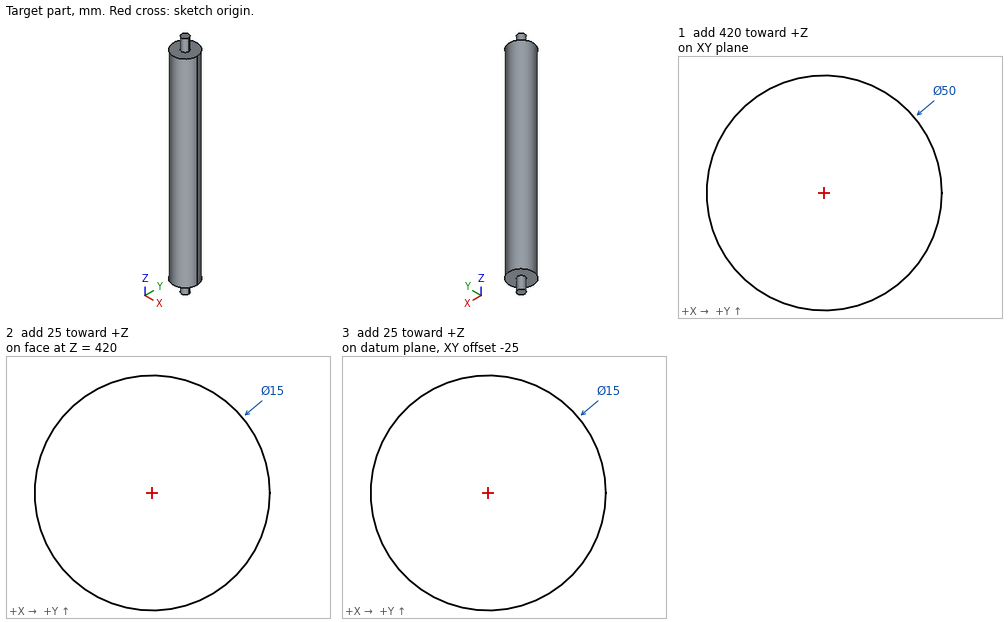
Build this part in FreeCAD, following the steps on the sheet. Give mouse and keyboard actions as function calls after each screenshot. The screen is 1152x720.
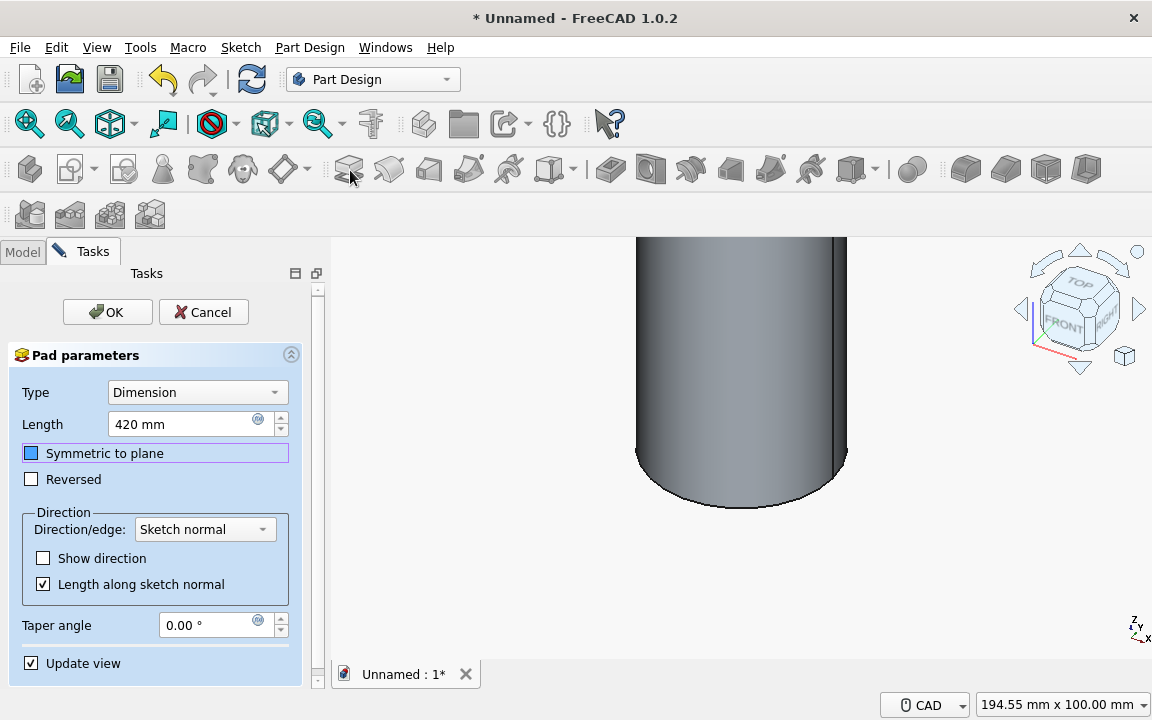
click(108, 312)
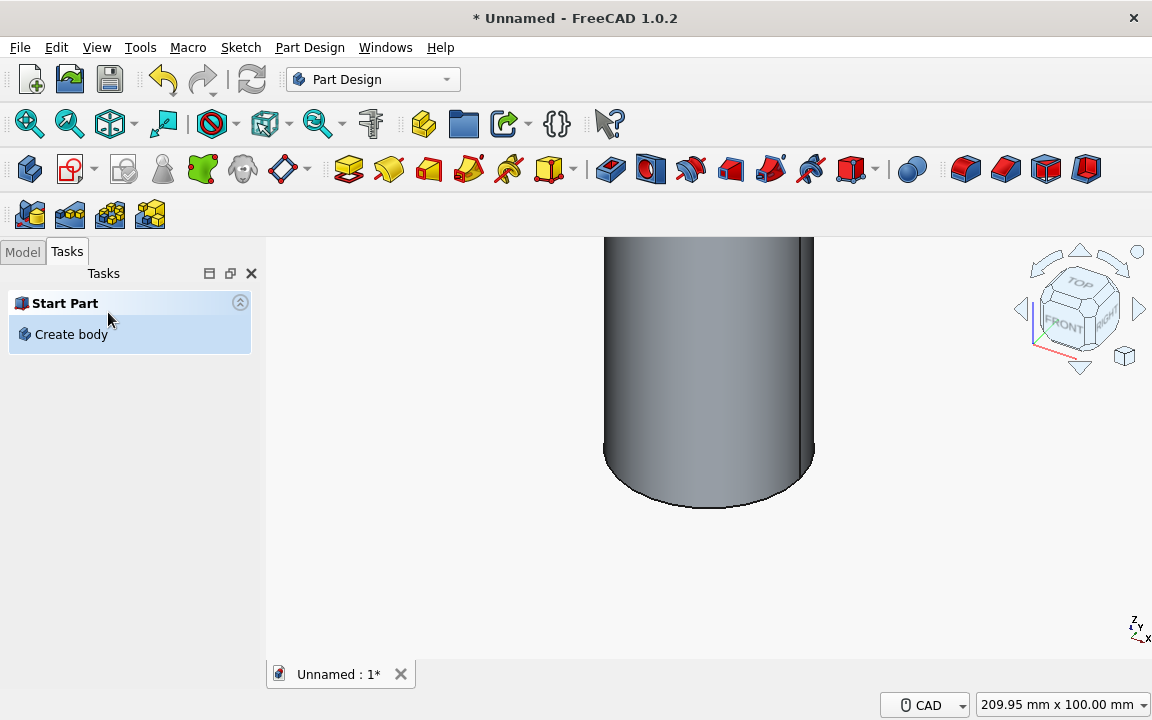
key(v)
key(f)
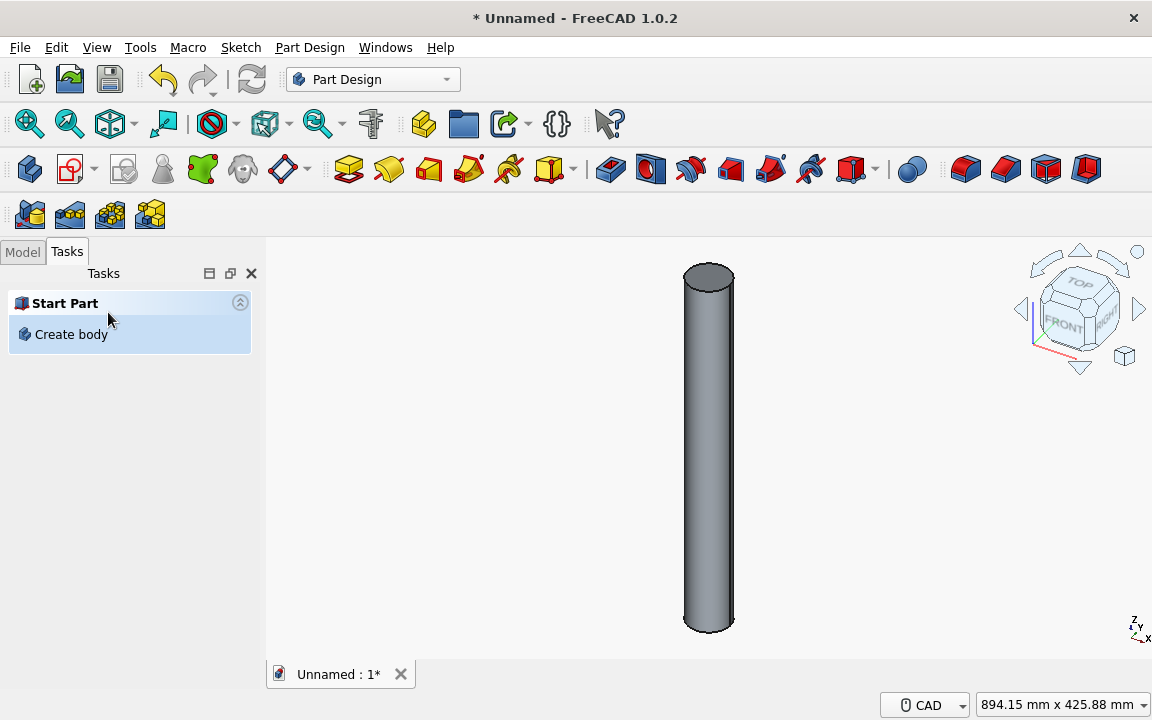
click(709, 277)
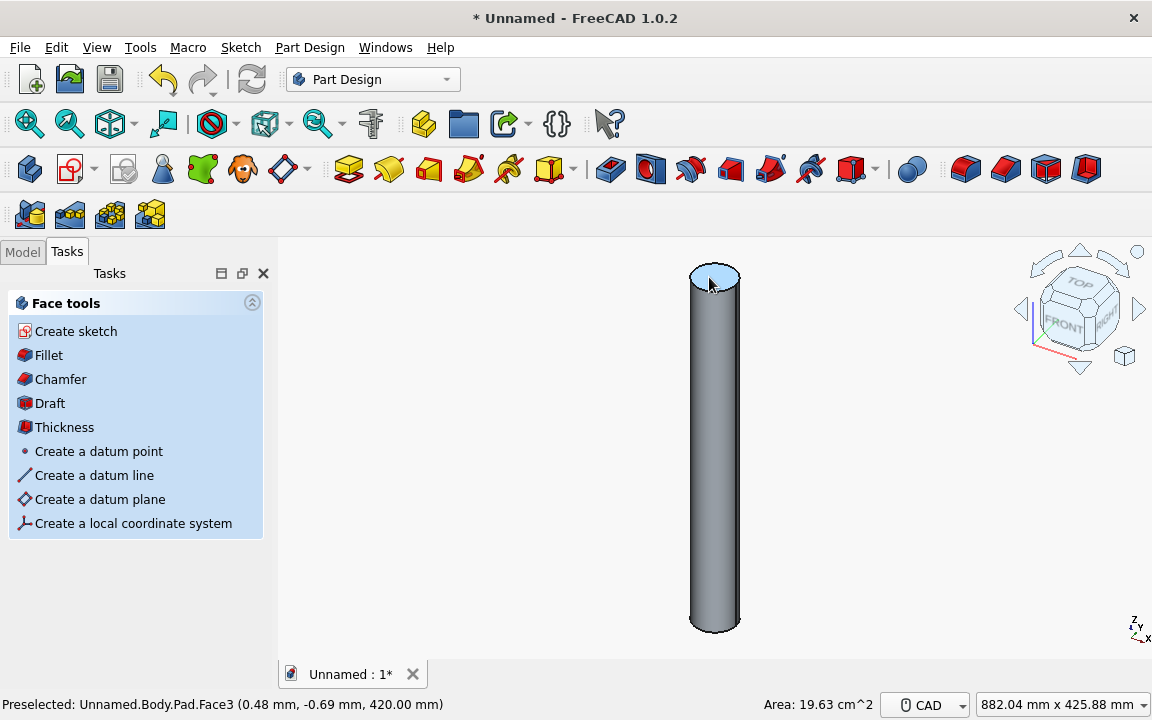
click(70, 170)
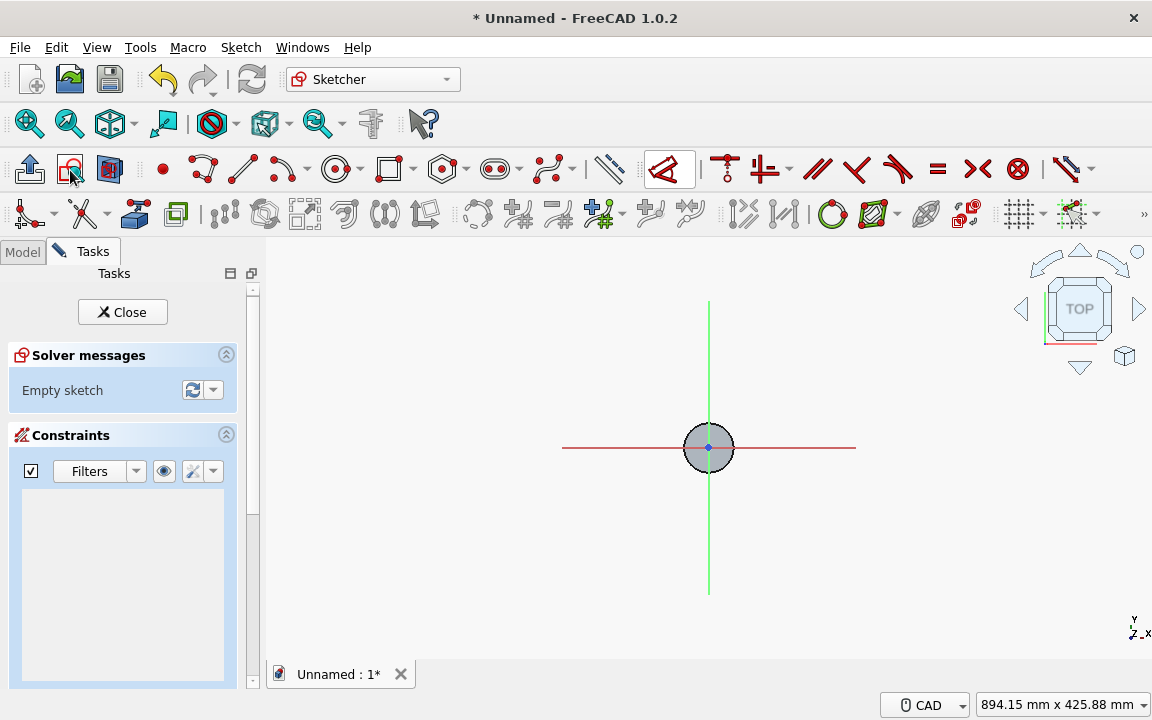
scroll(713, 448, up, 14)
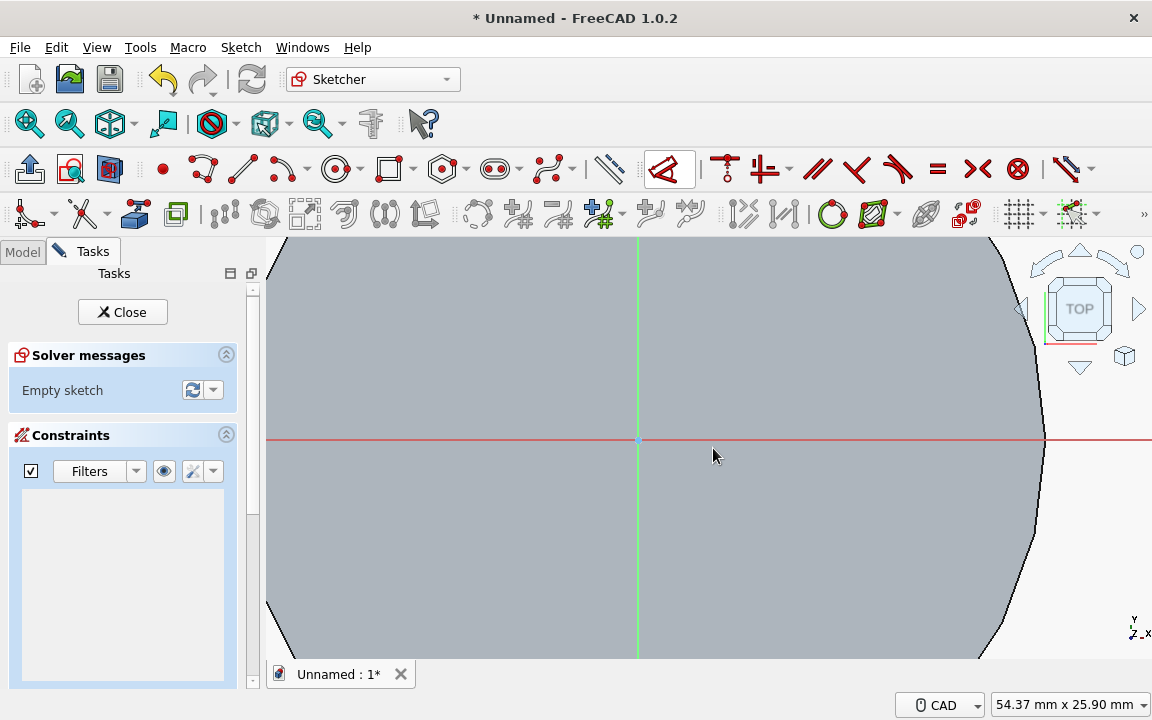
key(g)
key(c)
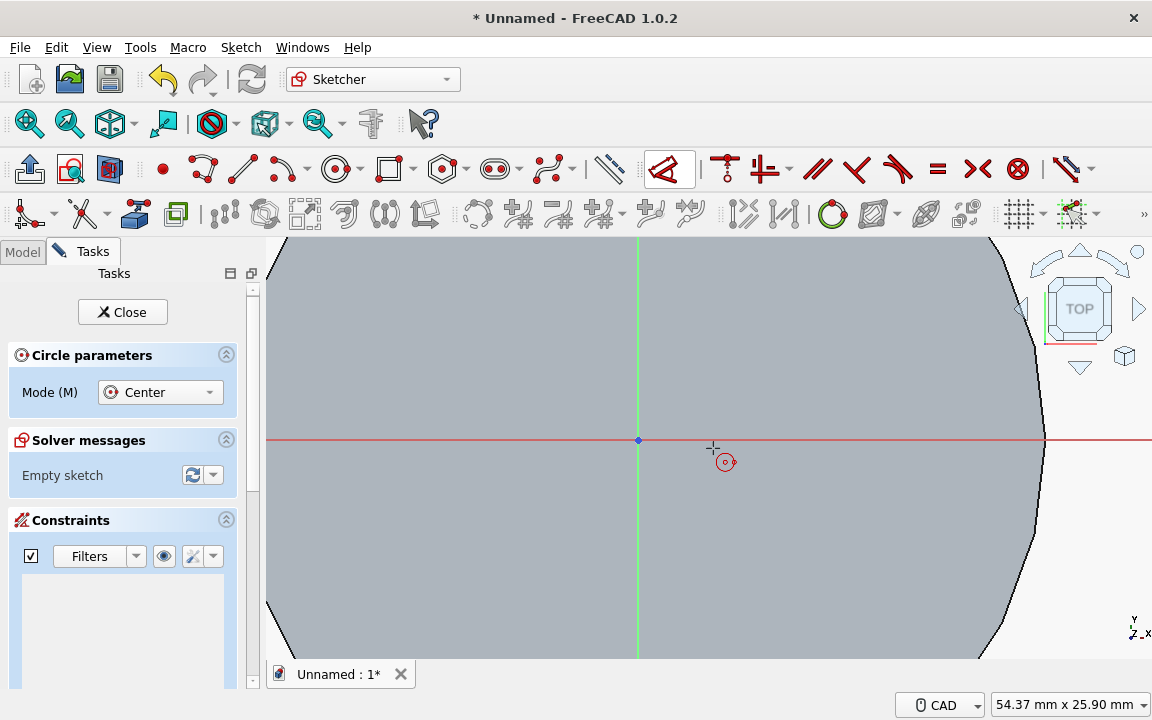
click(638, 440)
click(724, 354)
key(Escape)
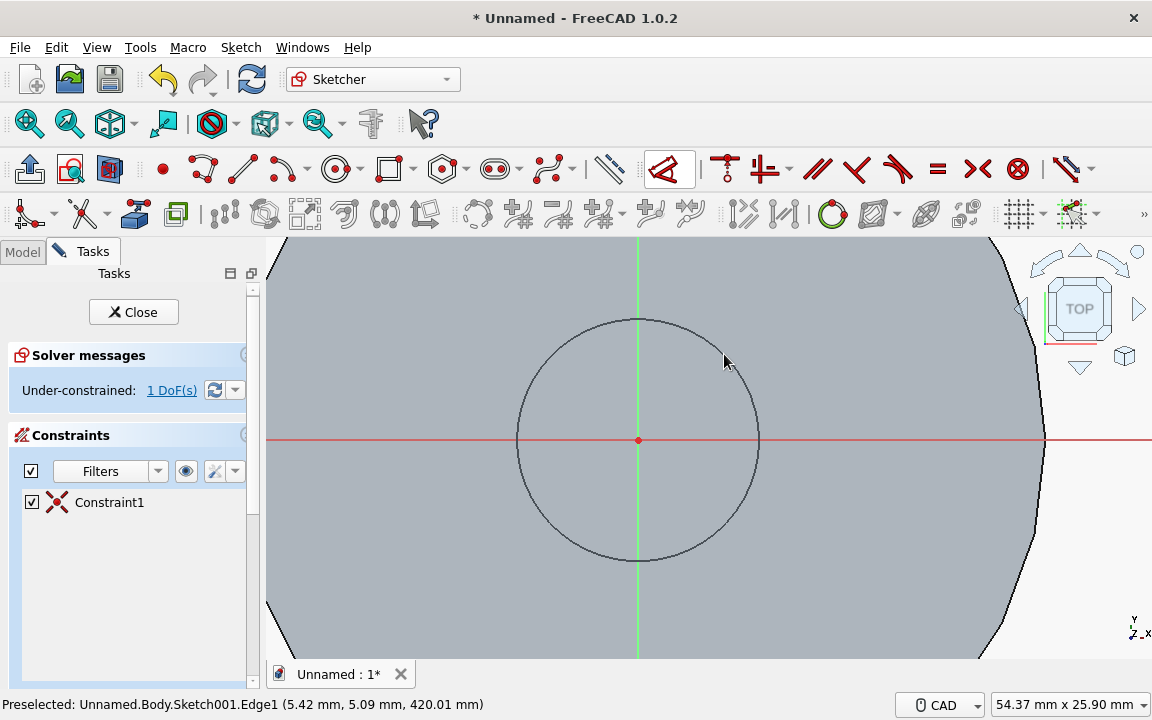
key(d)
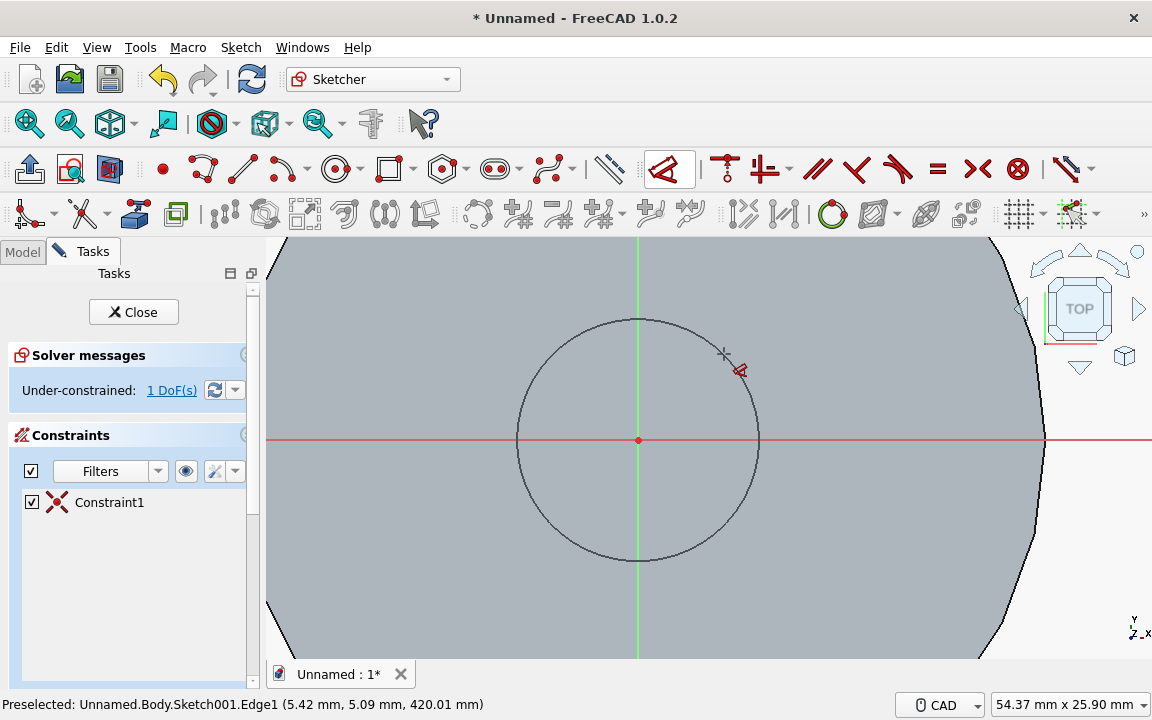
click(723, 354)
click(745, 331)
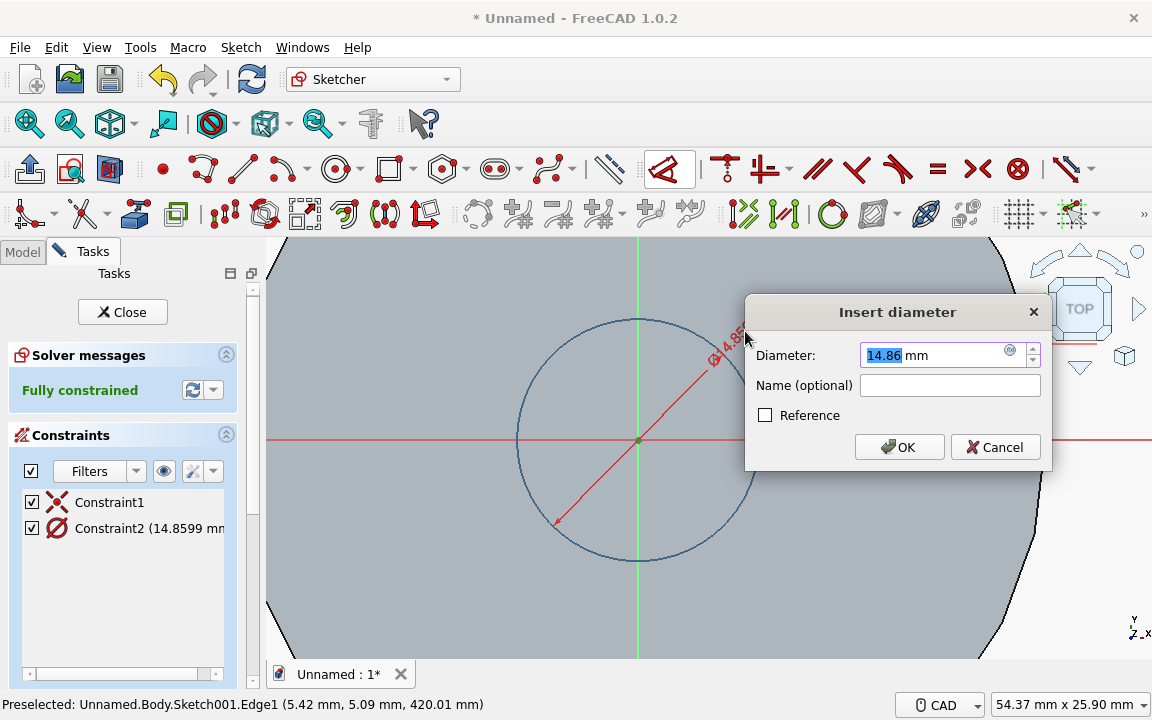
text(15)
key(Return)
key(Escape)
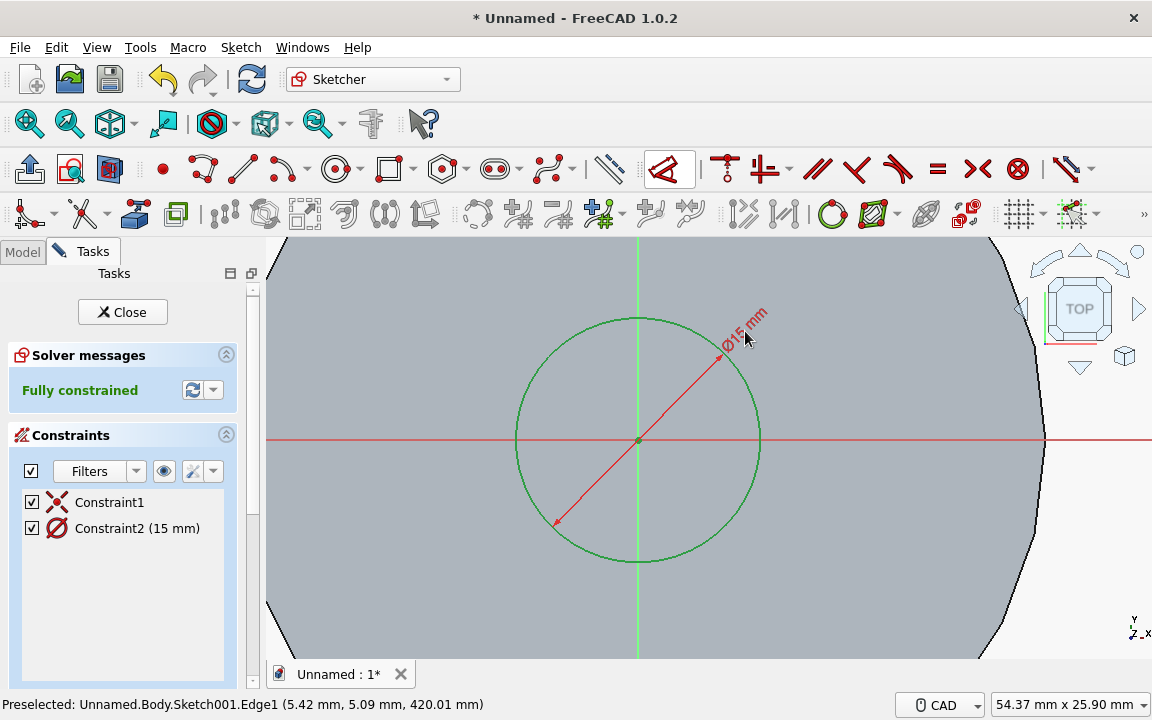
click(123, 312)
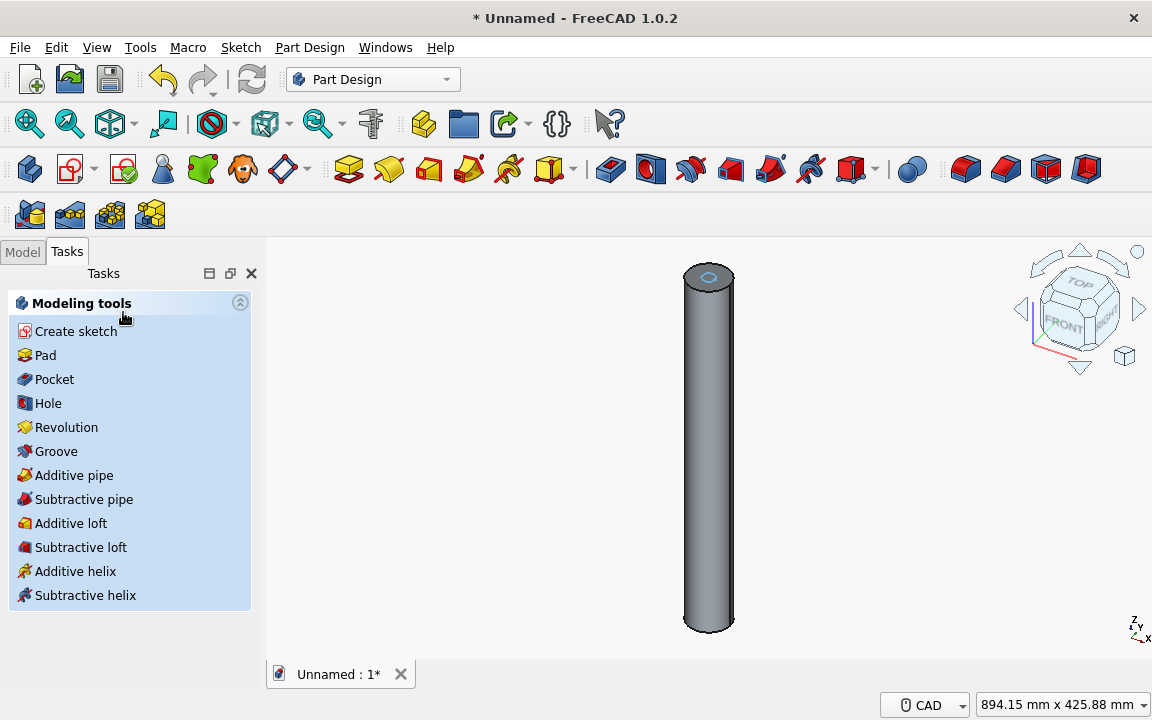
click(350, 170)